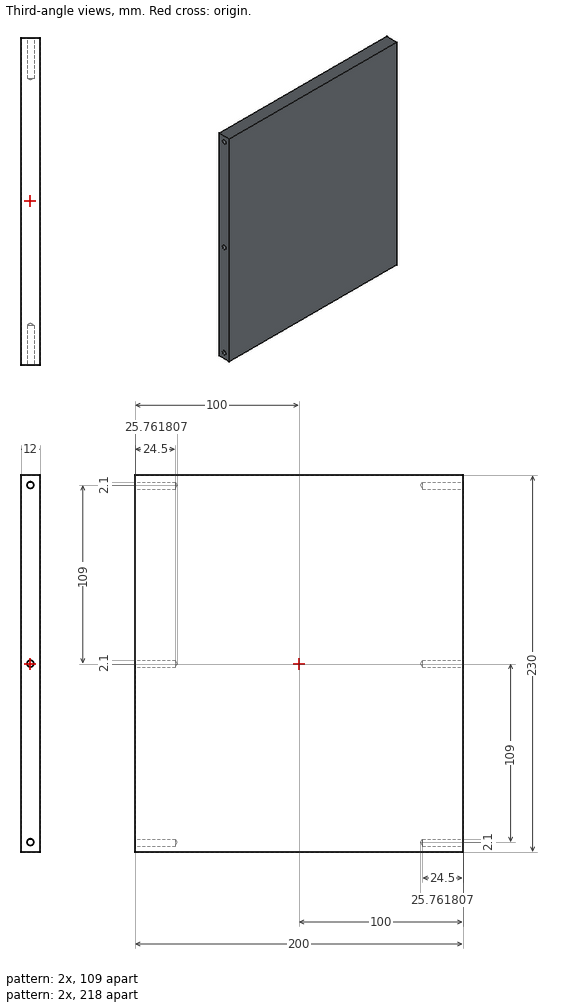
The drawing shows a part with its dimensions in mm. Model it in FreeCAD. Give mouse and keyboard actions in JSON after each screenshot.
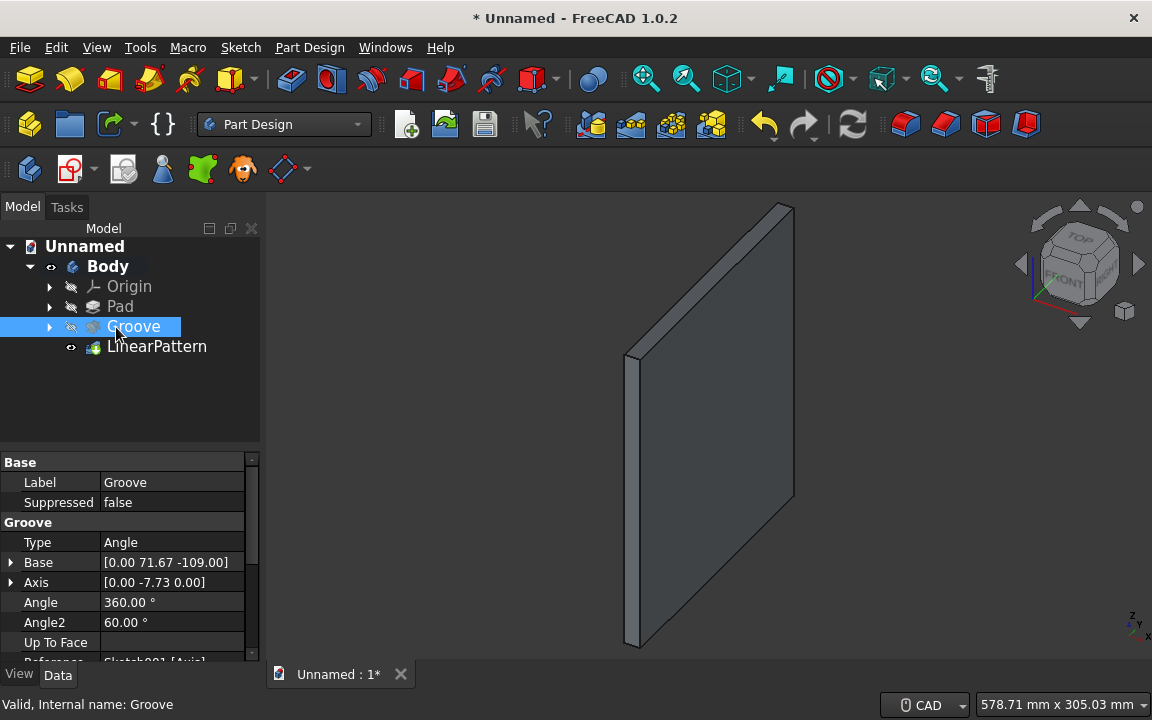
{"action": "left_click", "coordinate": [632, 124]}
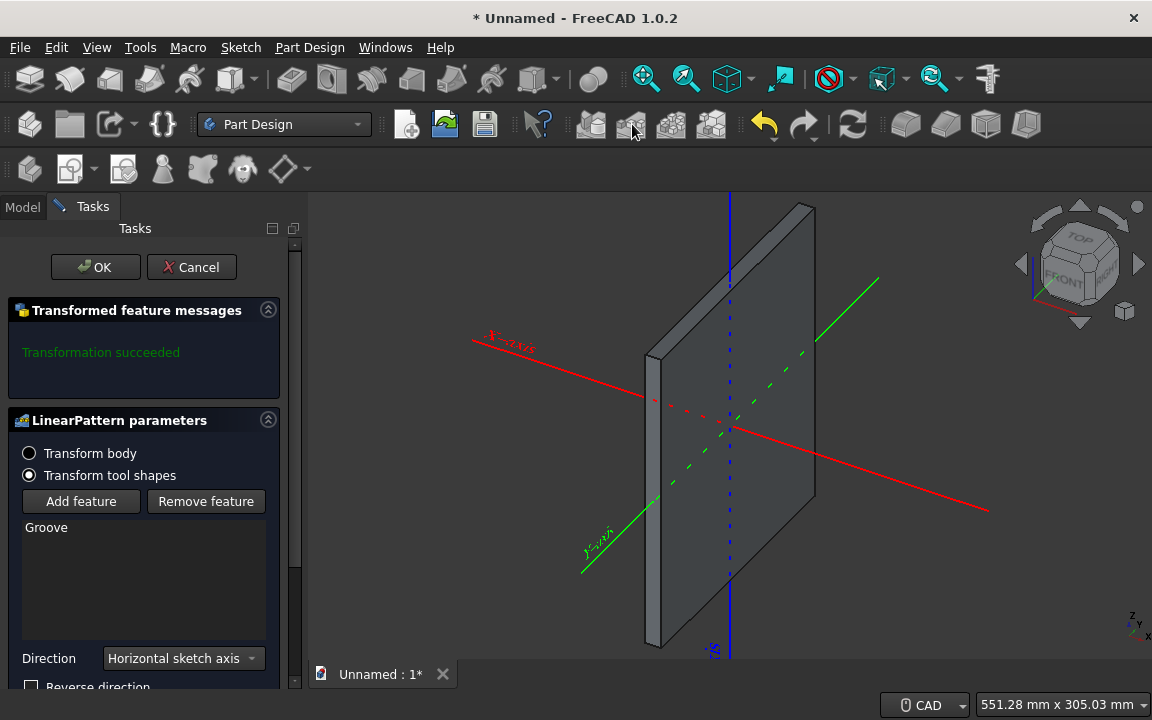
{"action": "left_click", "coordinate": [184, 658]}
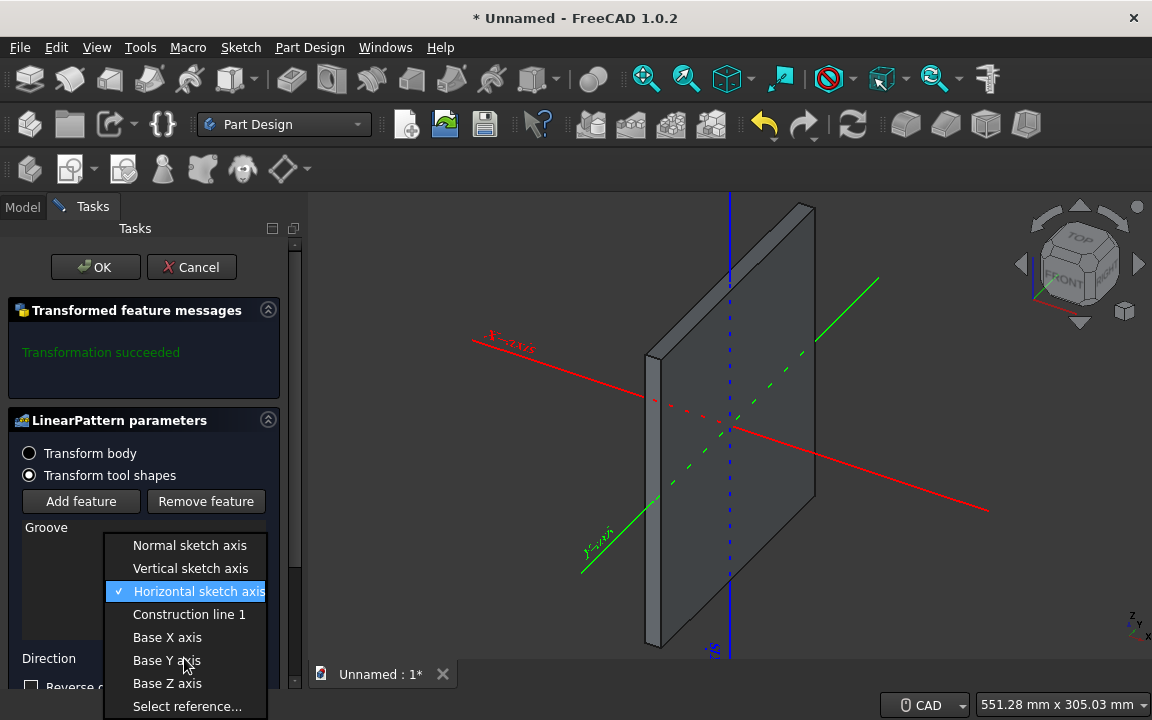
{"action": "left_click", "coordinate": [184, 684]}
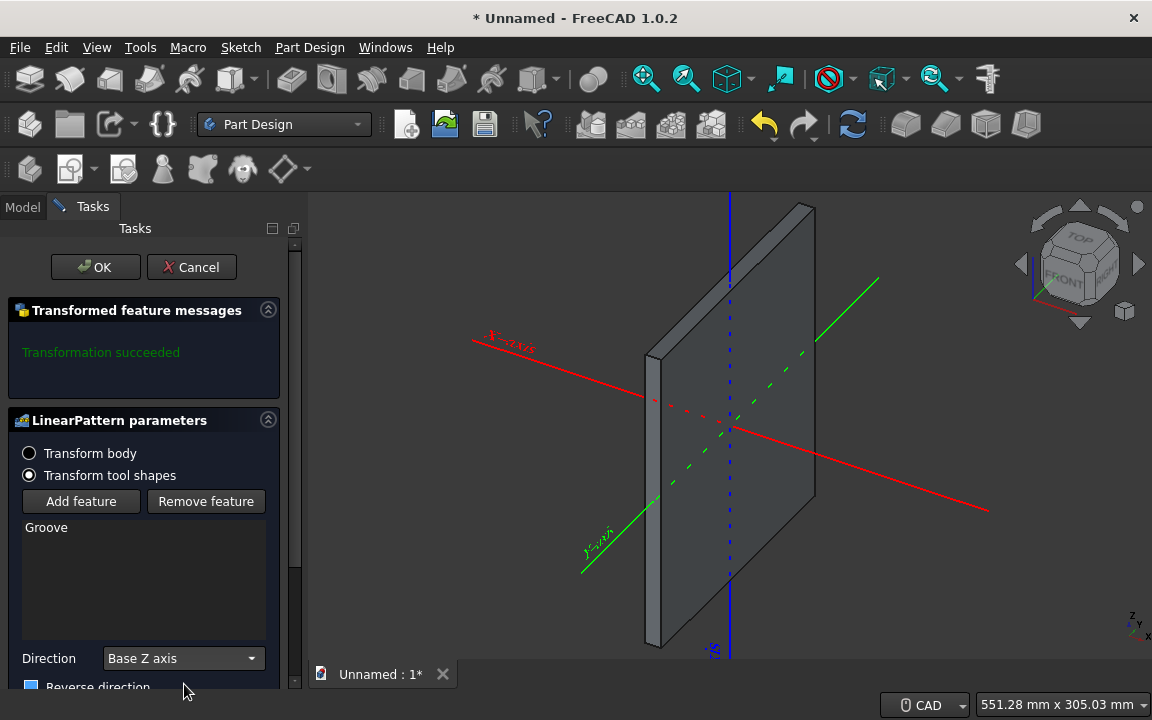
{"action": "scroll", "coordinate": [295, 463], "scroll_direction": "down", "scroll_amount": 2}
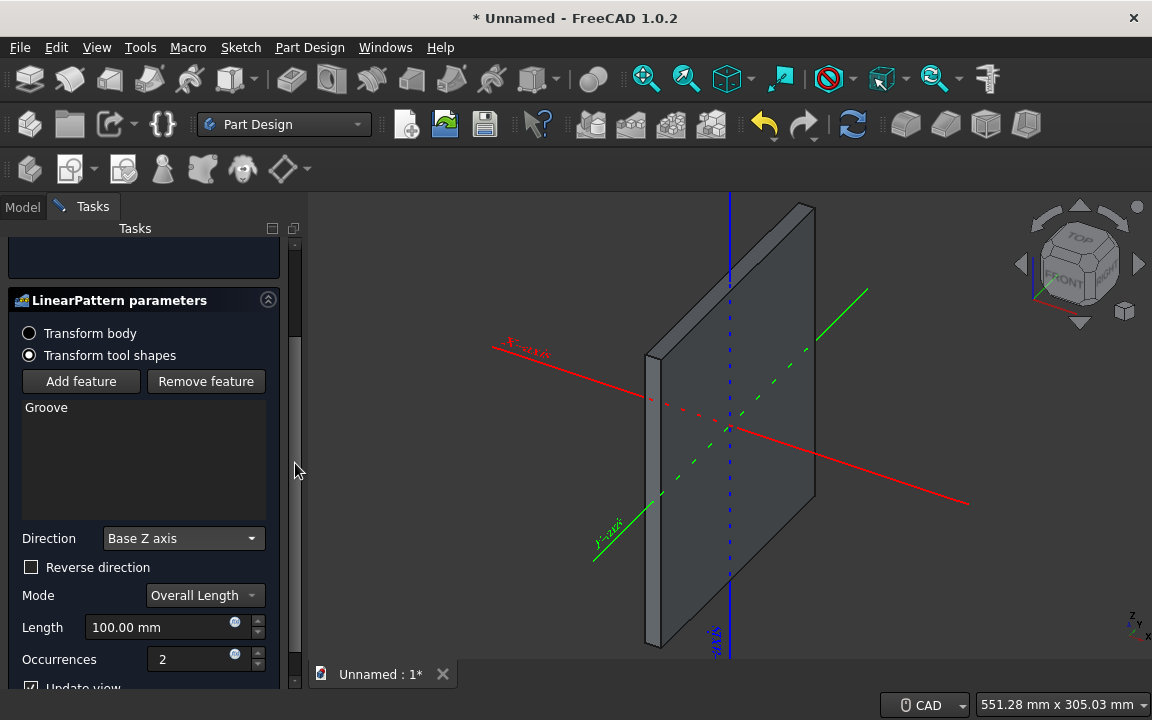
{"action": "left_click", "coordinate": [206, 596]}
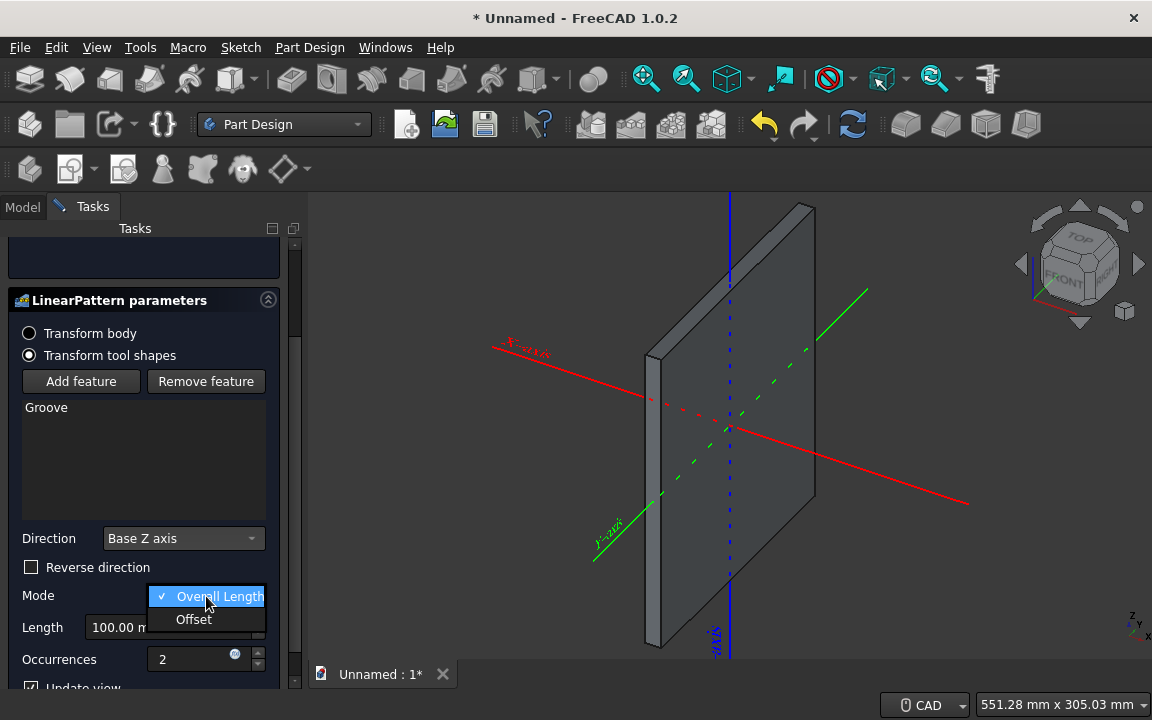
{"action": "left_click", "coordinate": [206, 620]}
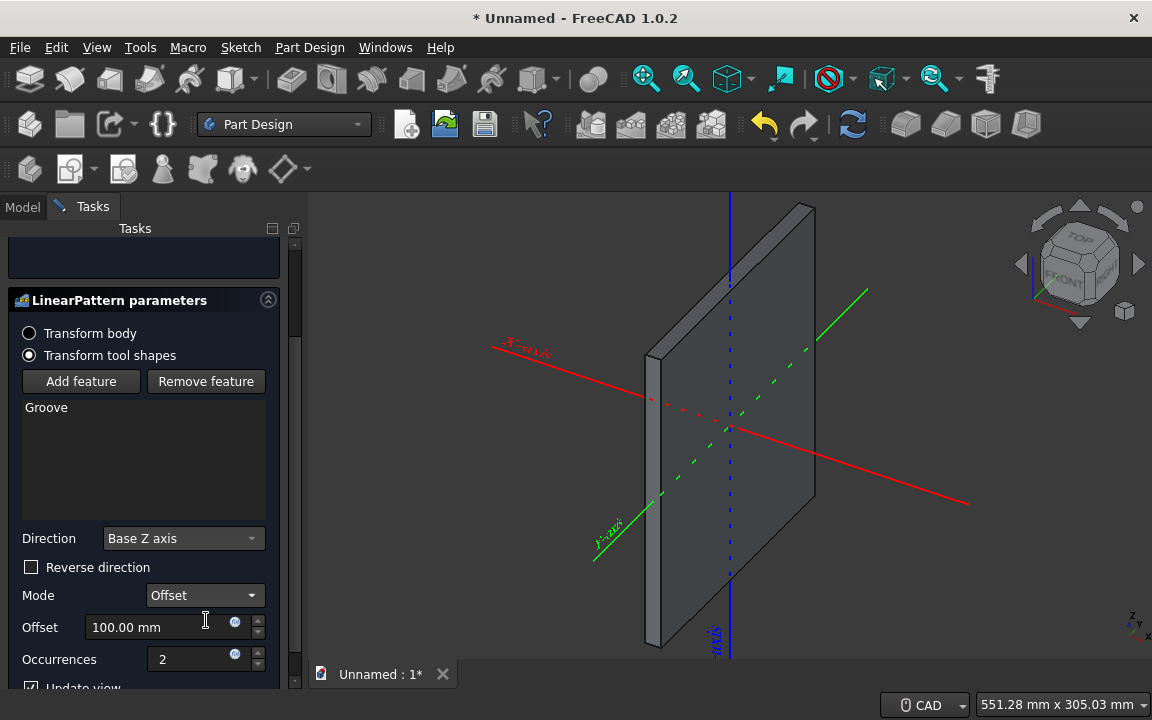
{"action": "triple_click", "coordinate": [168, 627]}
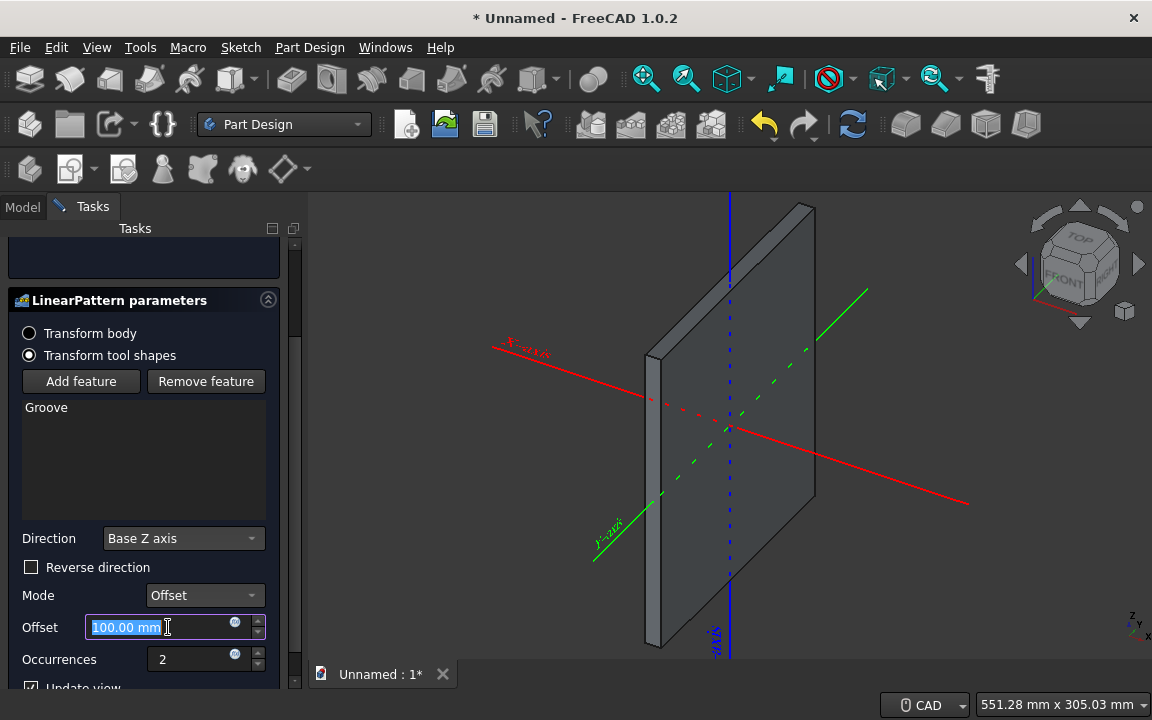
{"action": "type", "text": "218"}
{"action": "key", "text": "Tab"}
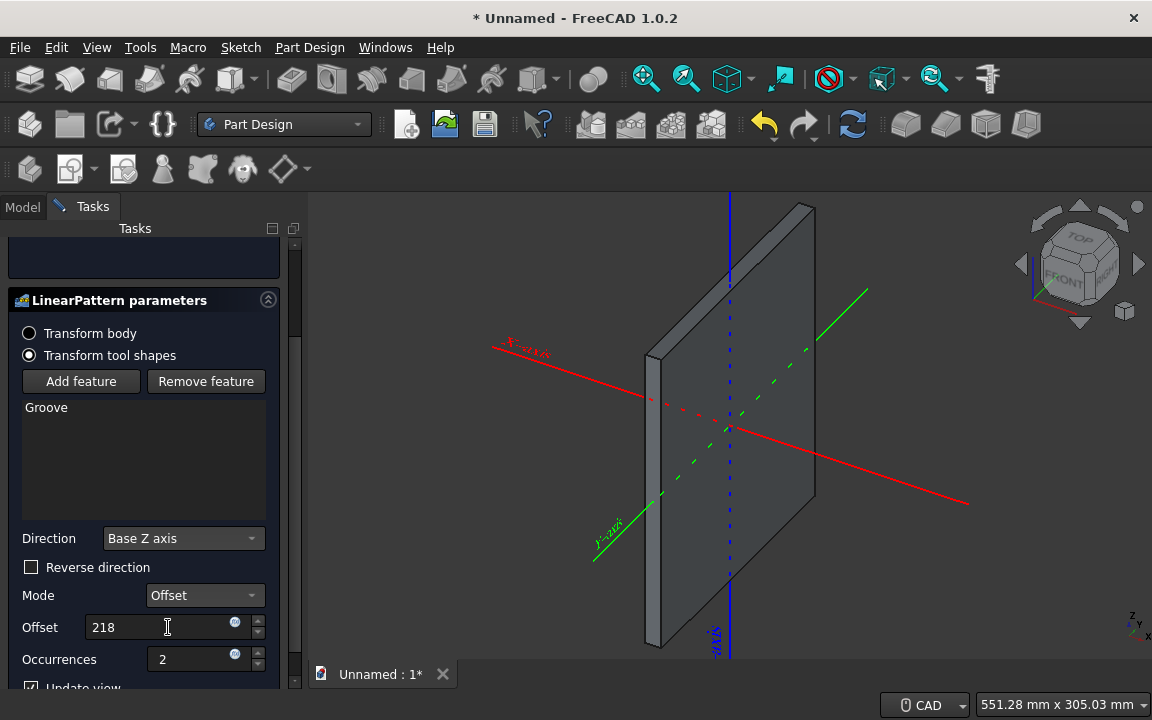
{"action": "triple_click", "coordinate": [198, 659]}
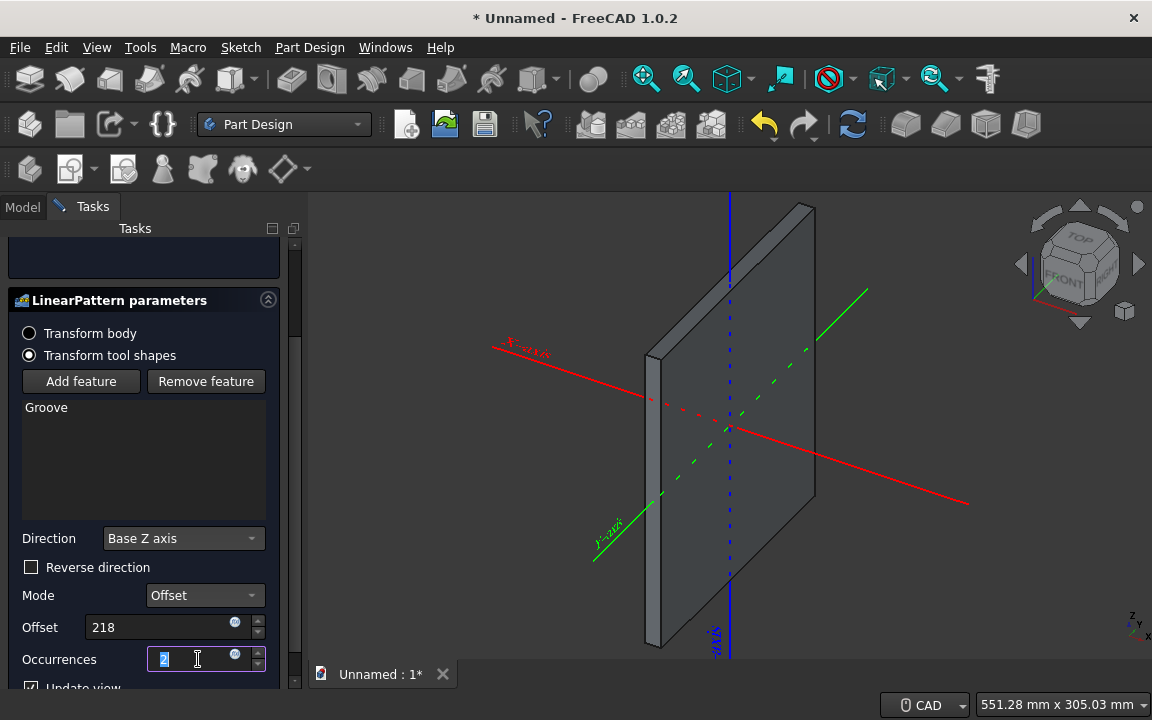
{"action": "type", "text": "2"}
{"action": "key", "text": "Tab"}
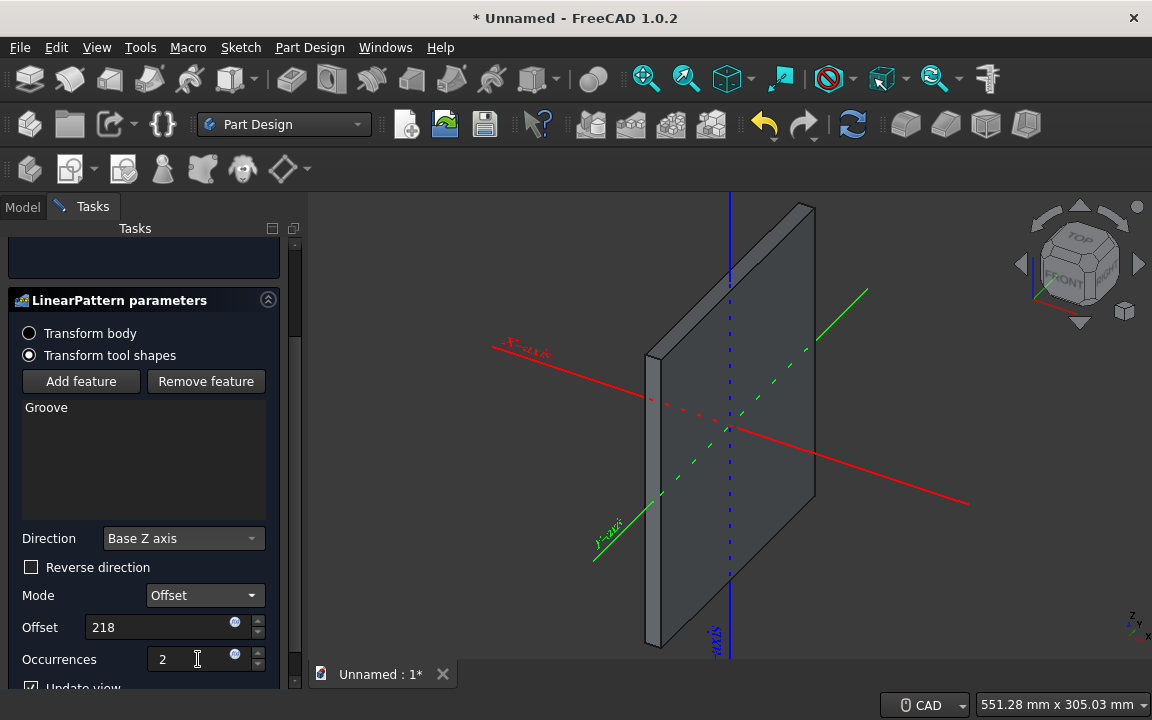
{"action": "scroll", "coordinate": [295, 463], "scroll_direction": "up", "scroll_amount": 3}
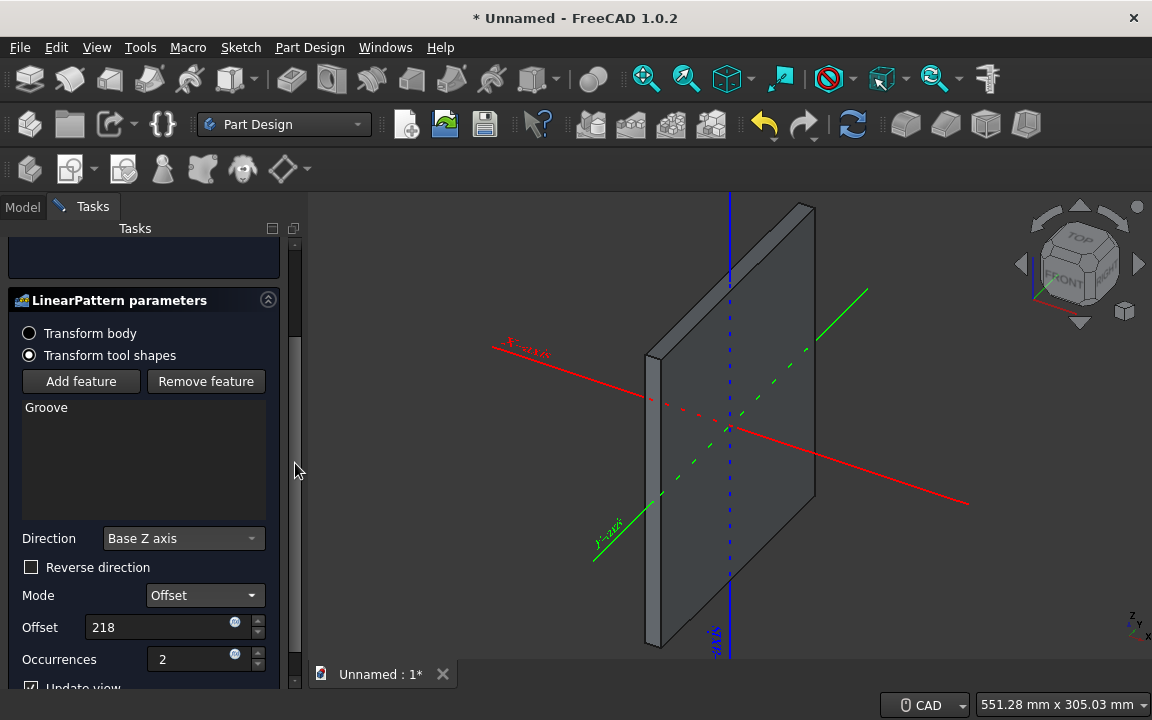
{"action": "left_click", "coordinate": [96, 267]}